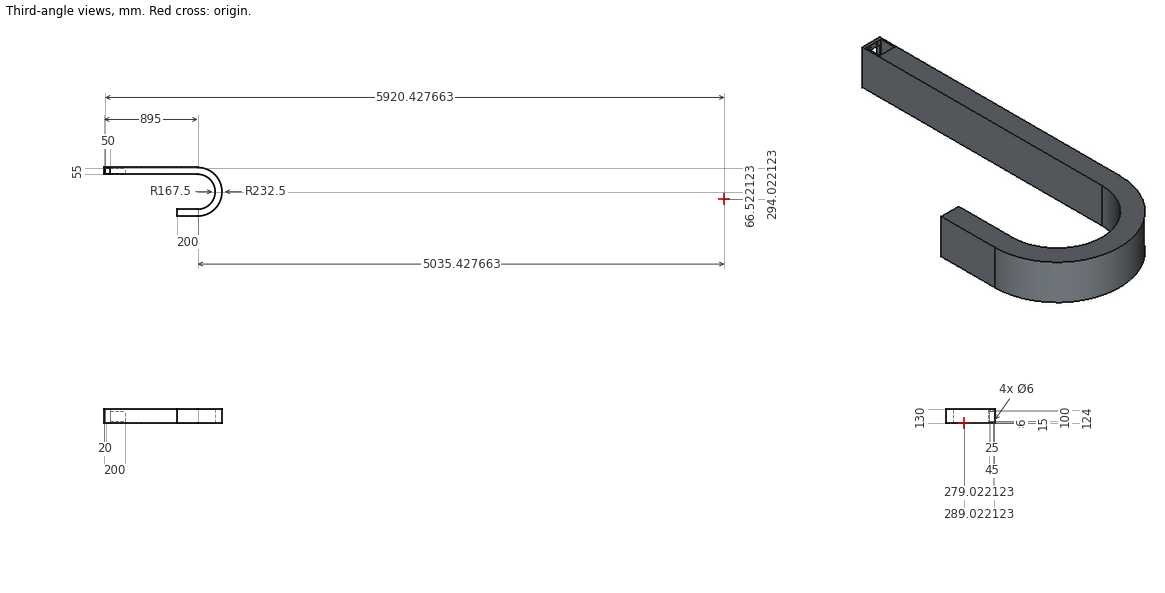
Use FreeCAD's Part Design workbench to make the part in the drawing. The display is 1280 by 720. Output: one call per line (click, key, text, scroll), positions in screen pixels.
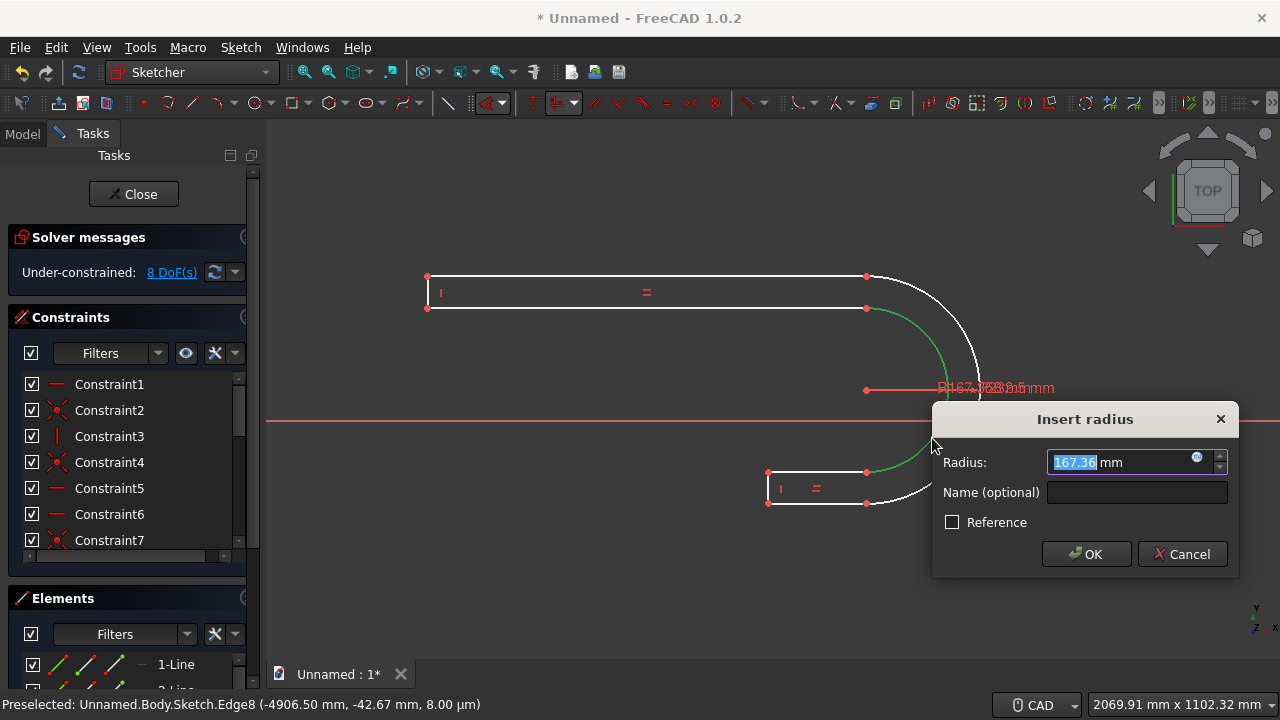
text(167.5)
key(Return)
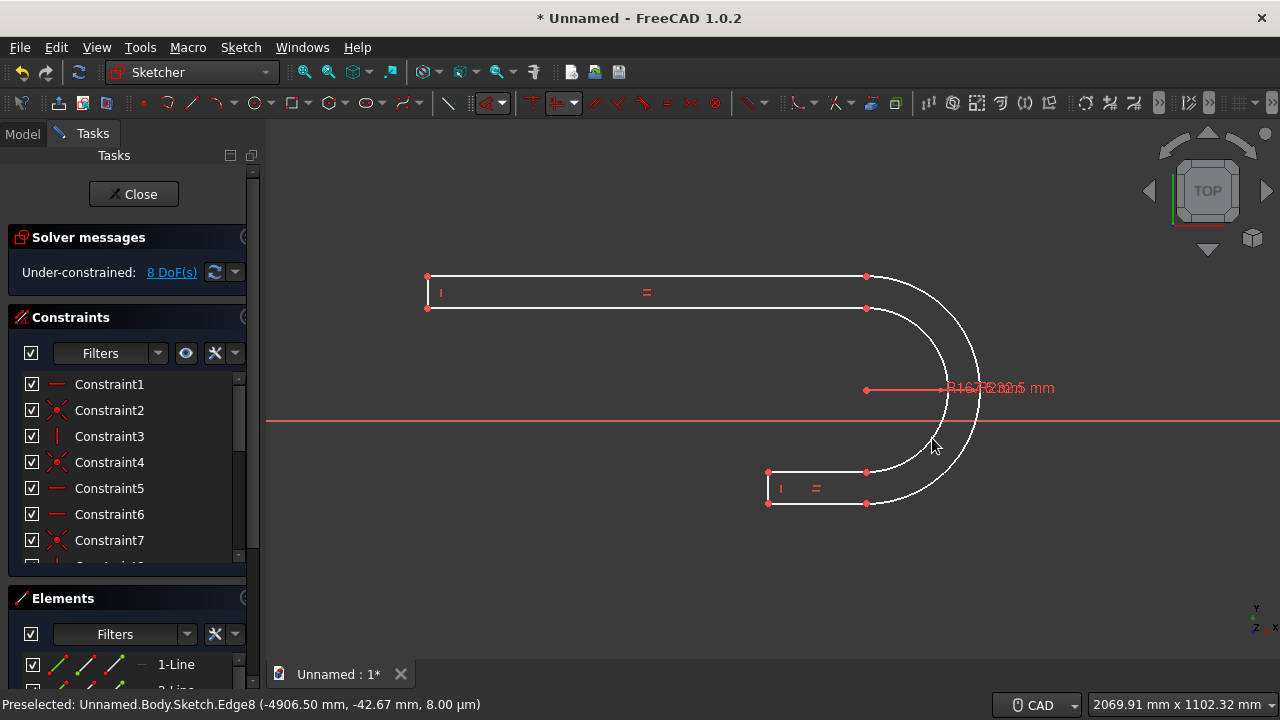
click(837, 472)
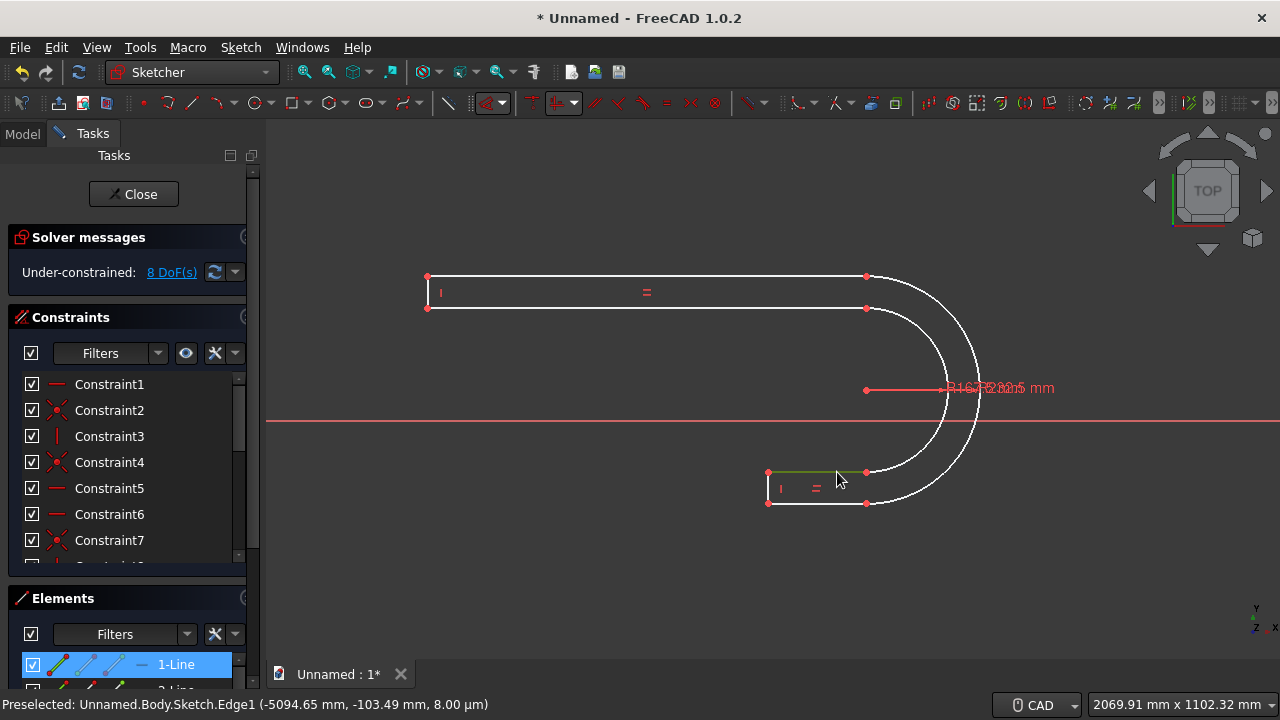
key(l)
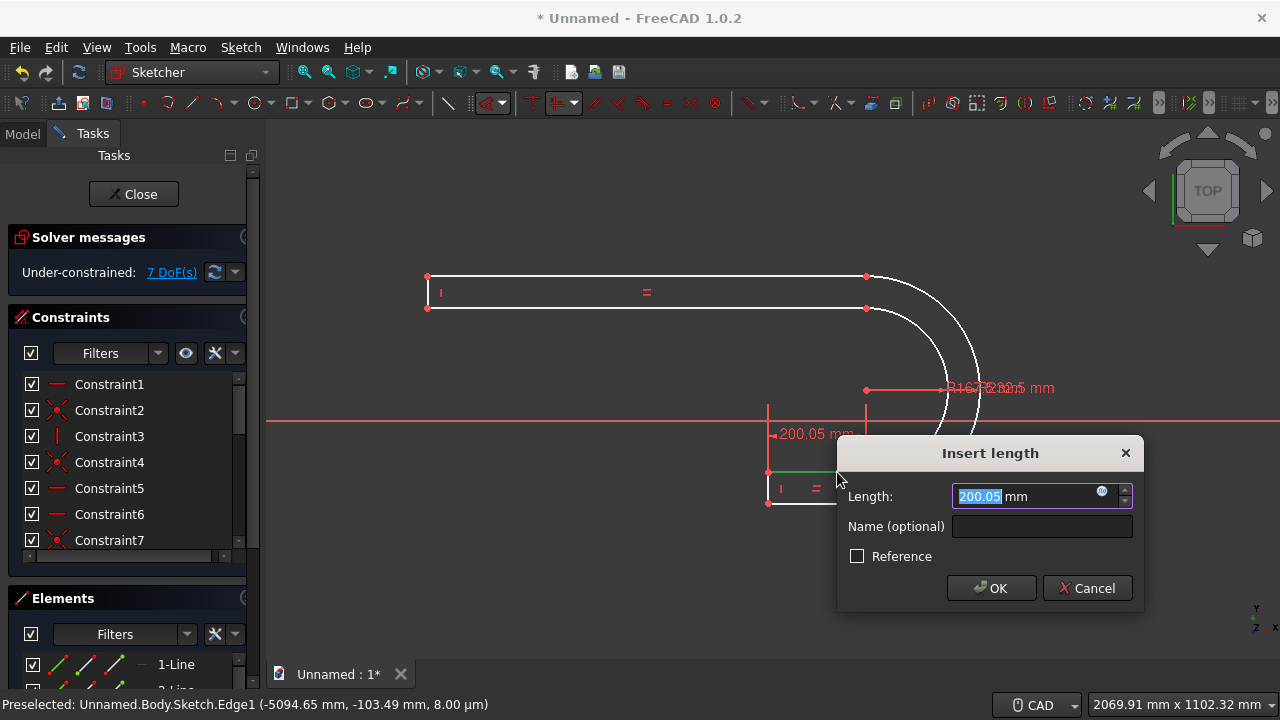
text(200)
key(Return)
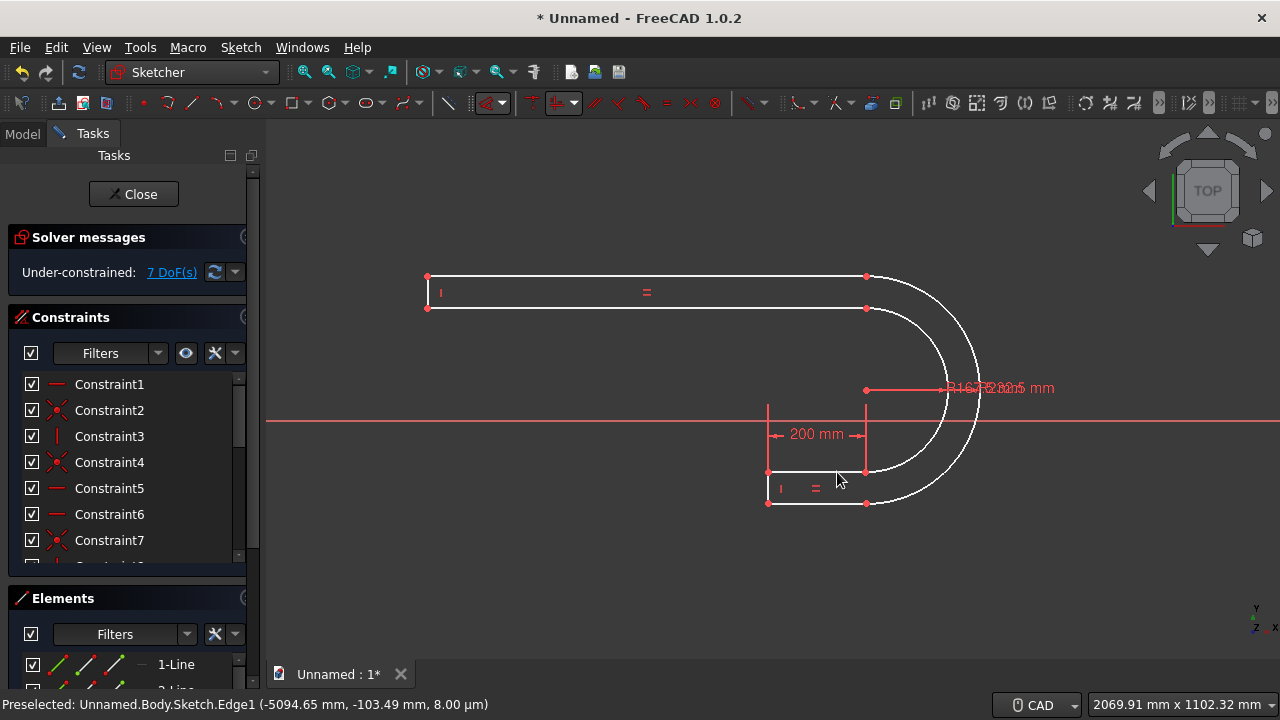
click(797, 504)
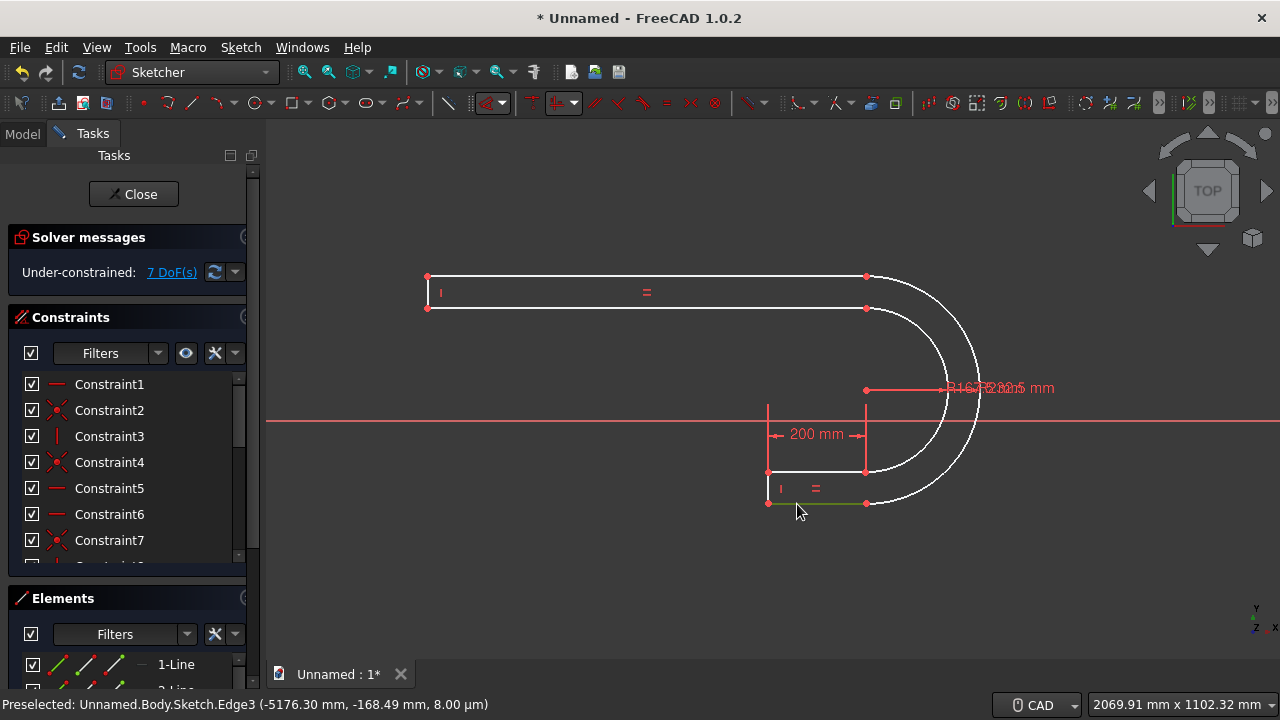
click(504, 104)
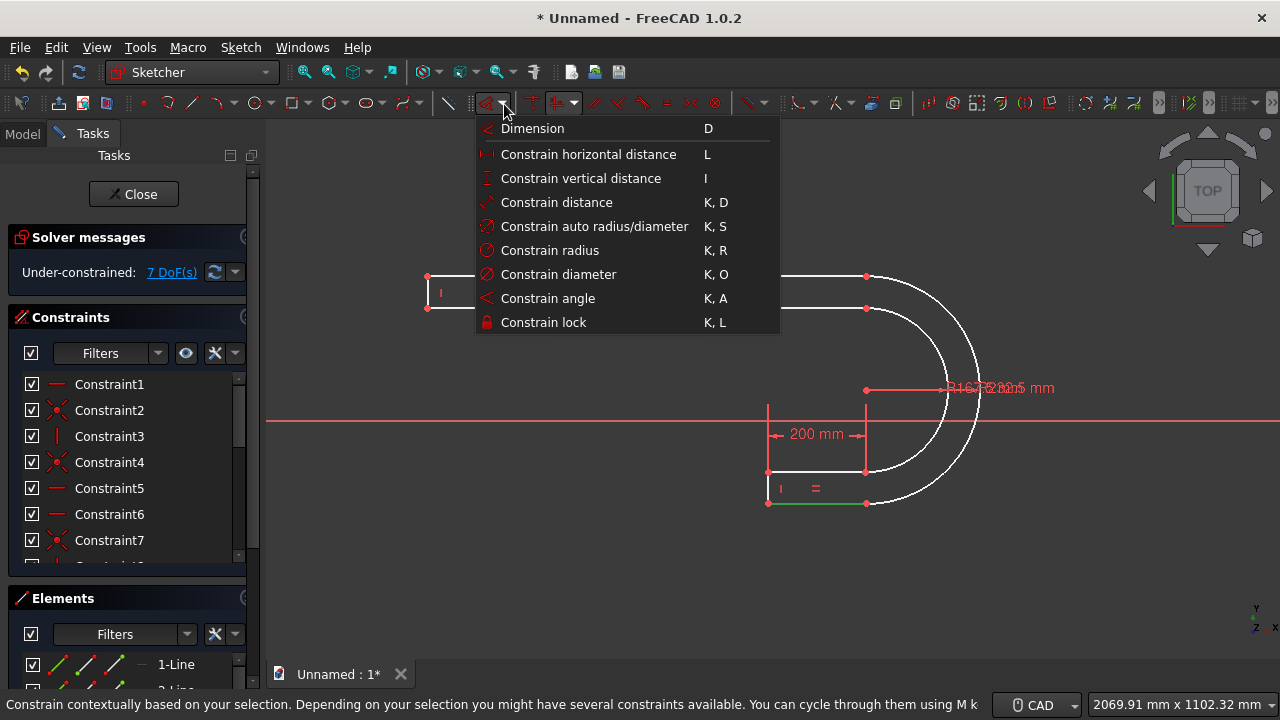
click(628, 154)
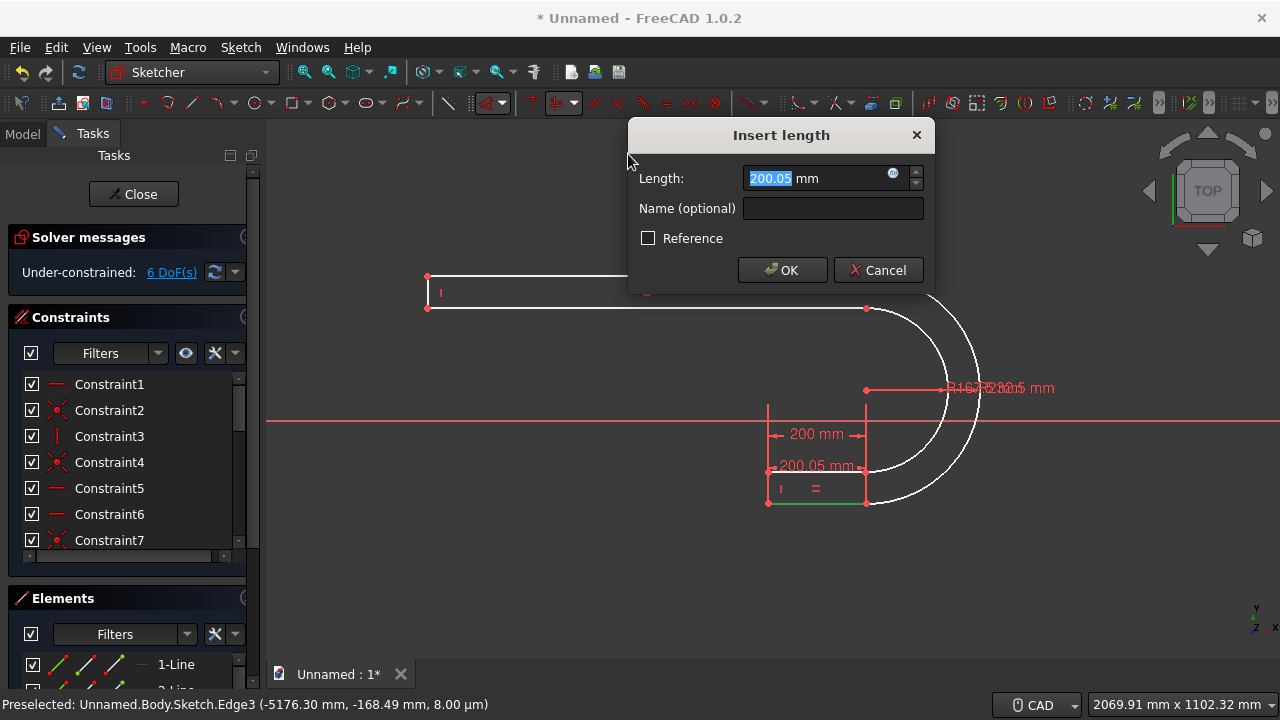
text(200)
key(Return)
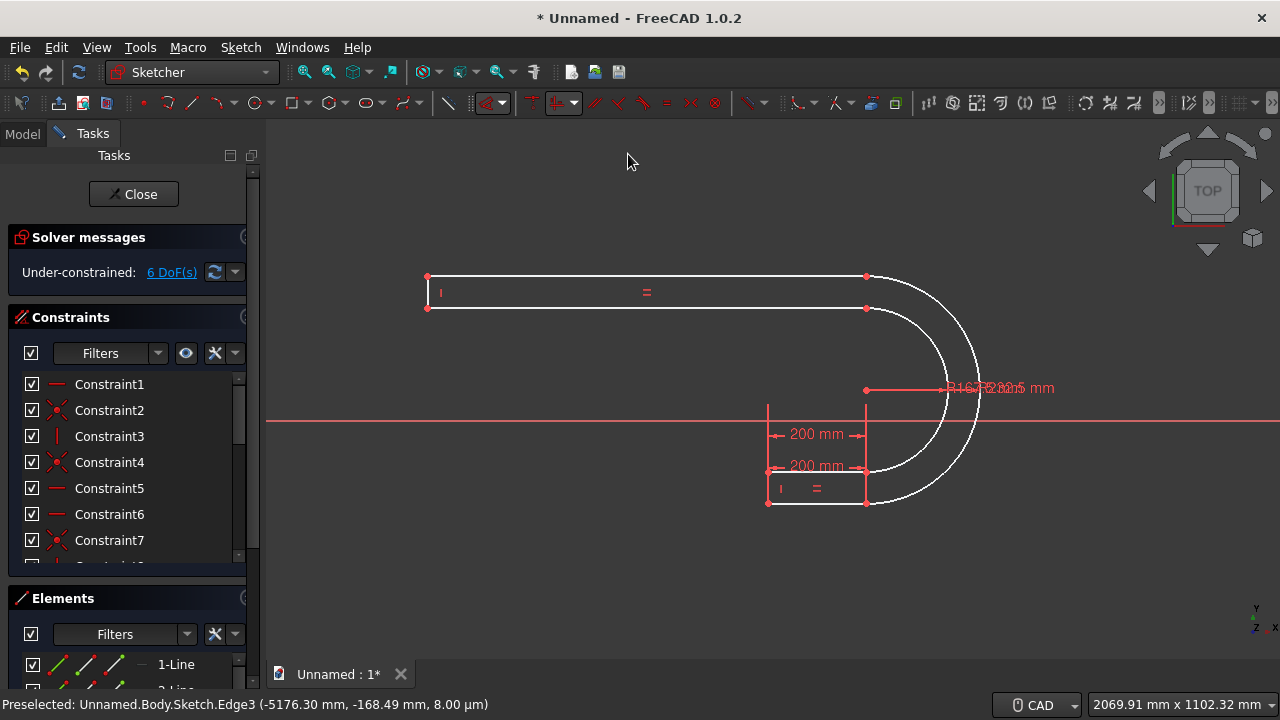
click(735, 276)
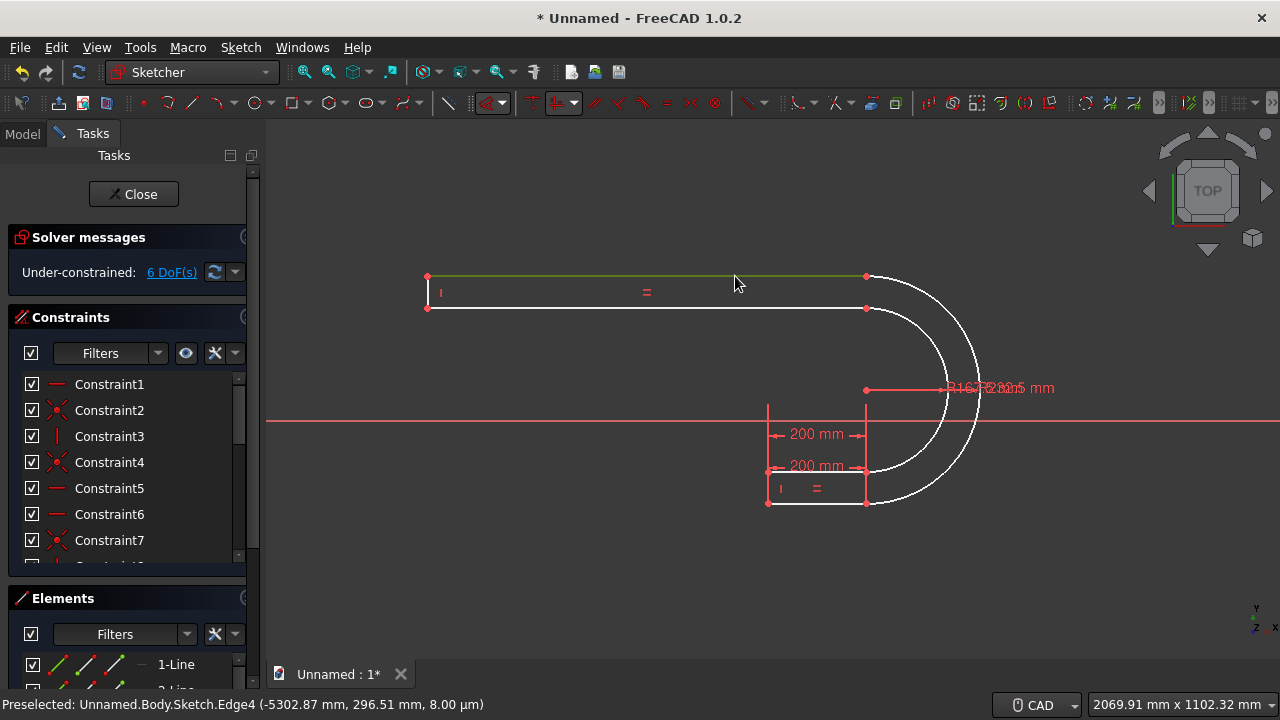
key(l)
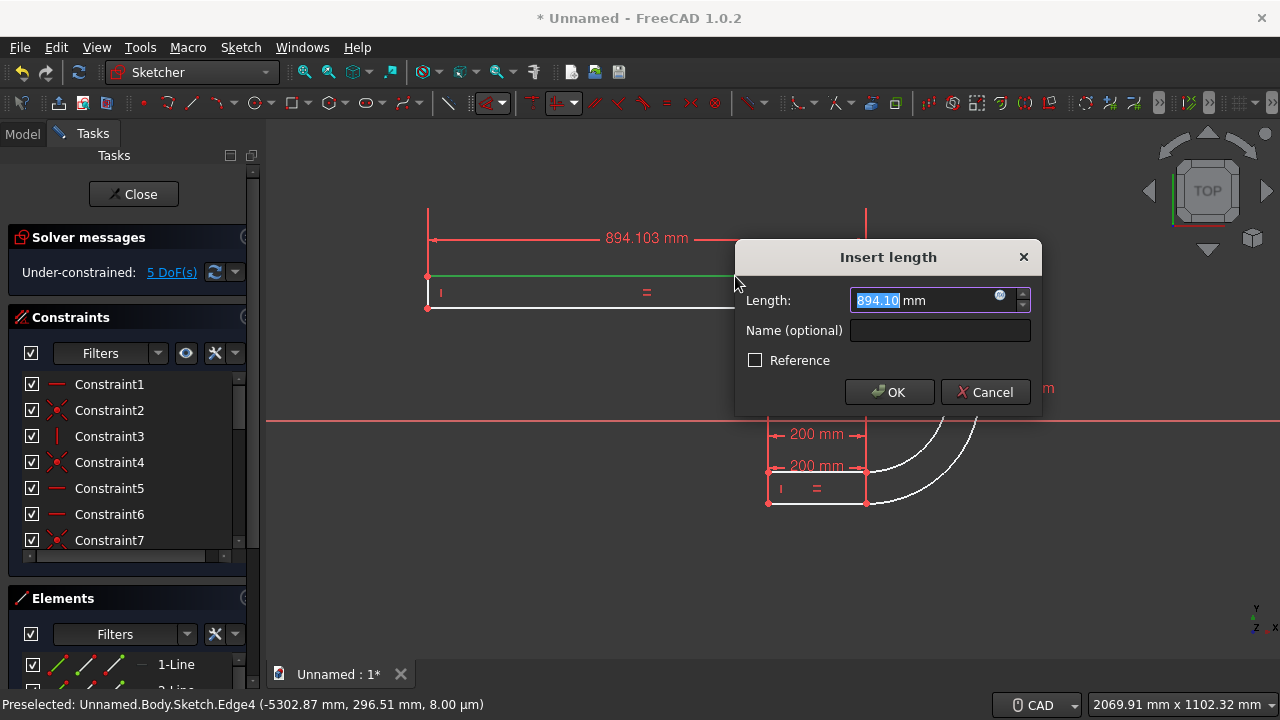
text(895)
key(Return)